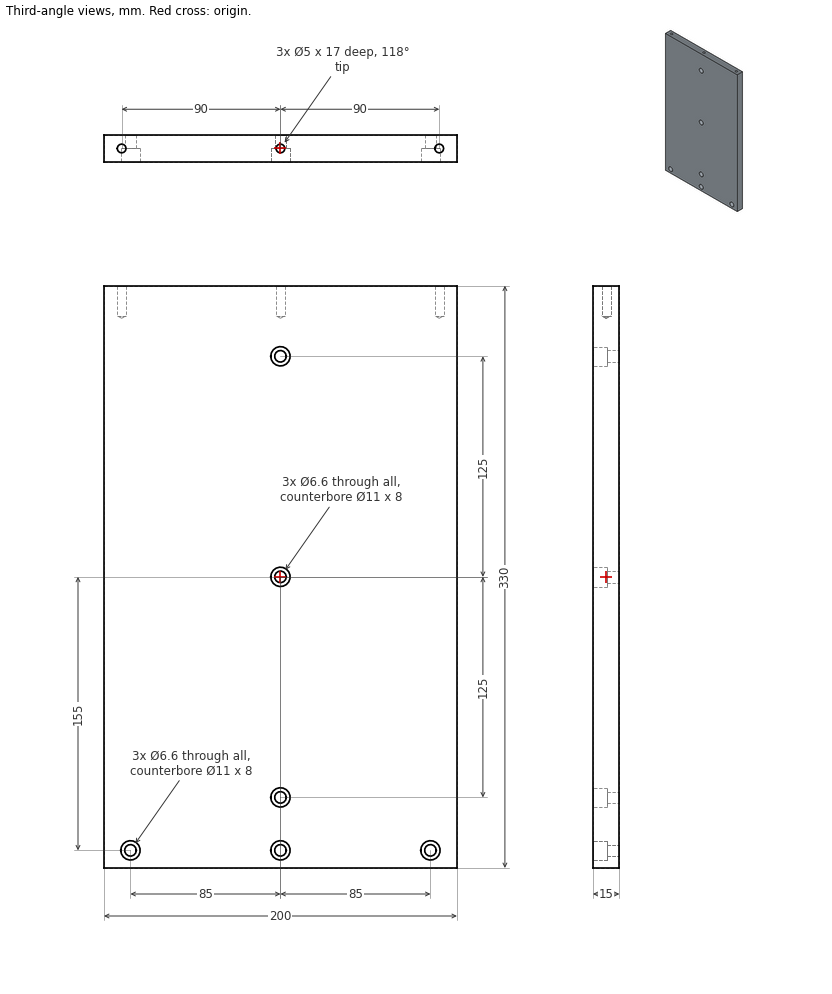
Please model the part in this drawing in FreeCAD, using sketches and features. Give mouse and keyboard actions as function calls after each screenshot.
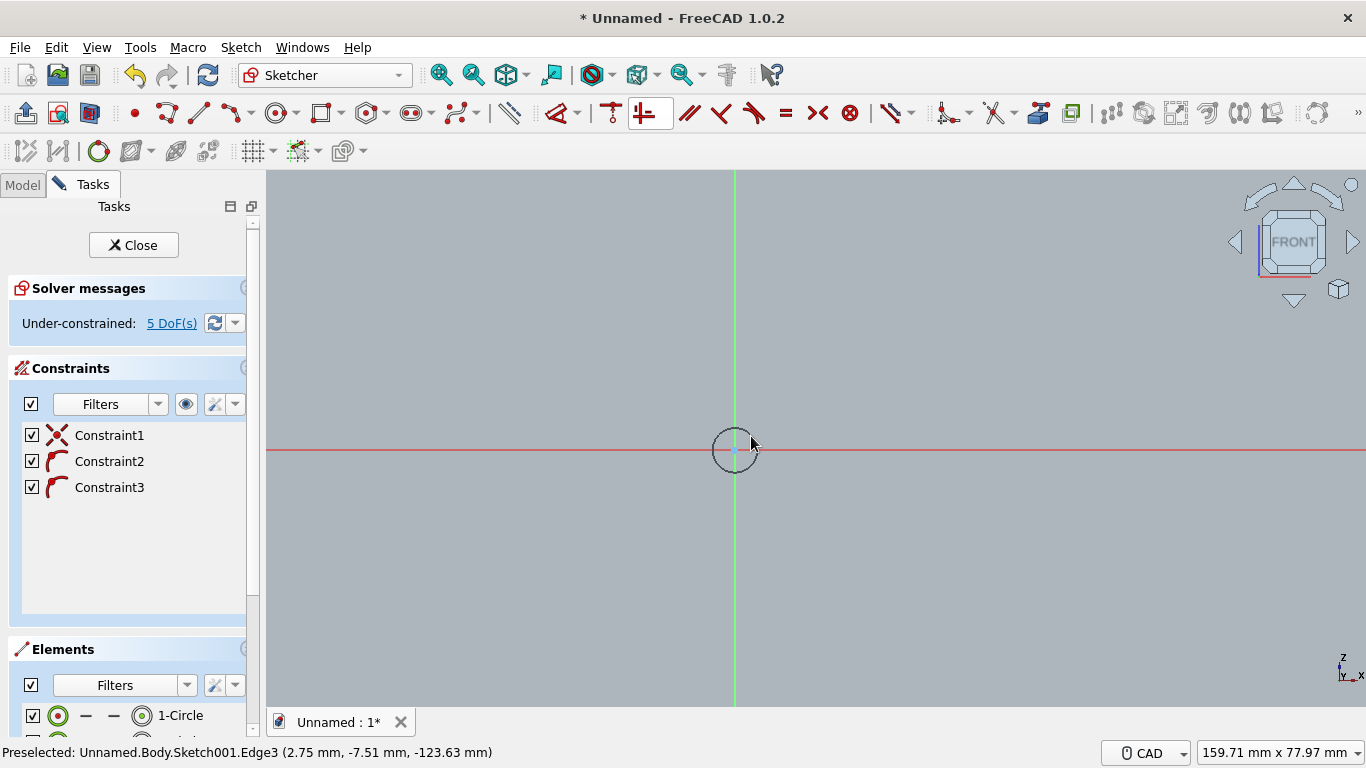
click(751, 435)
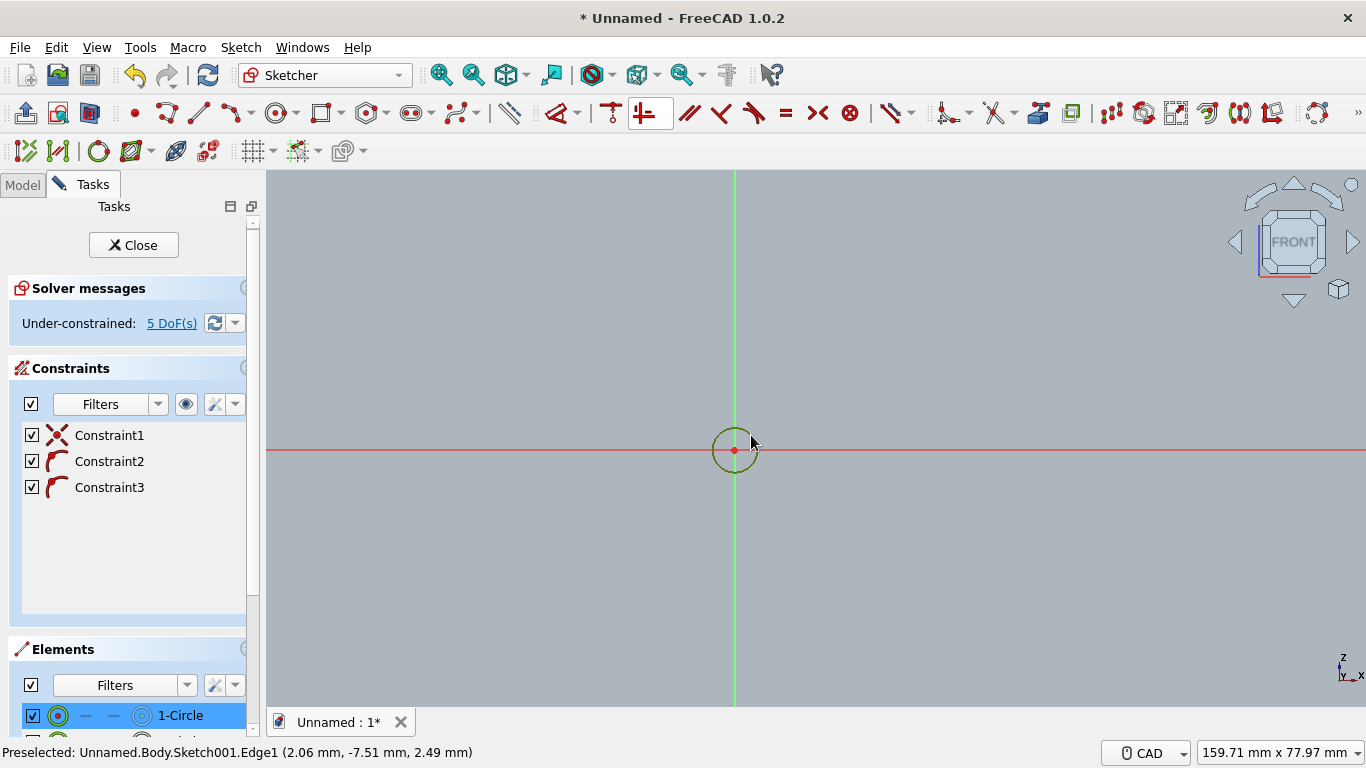
scroll(751, 435, down, 8)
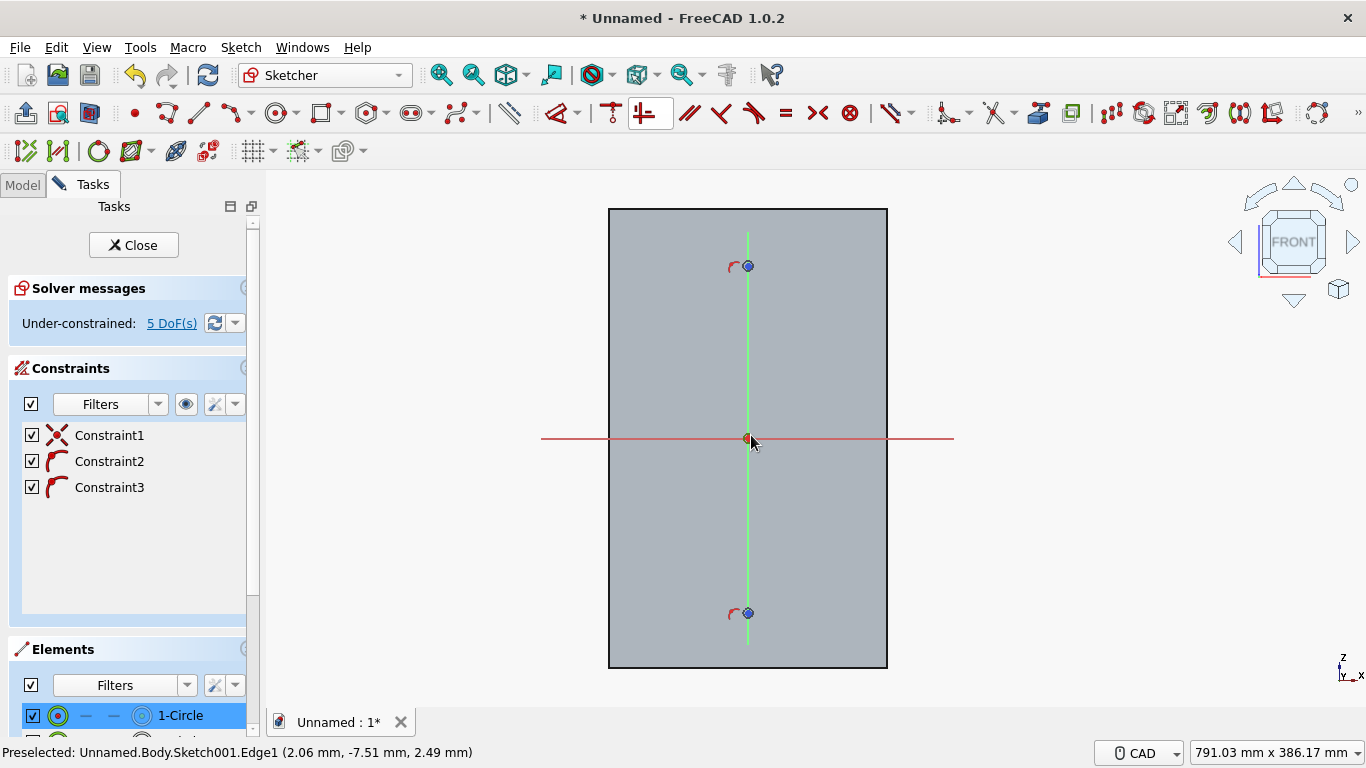
scroll(752, 262, up, 7)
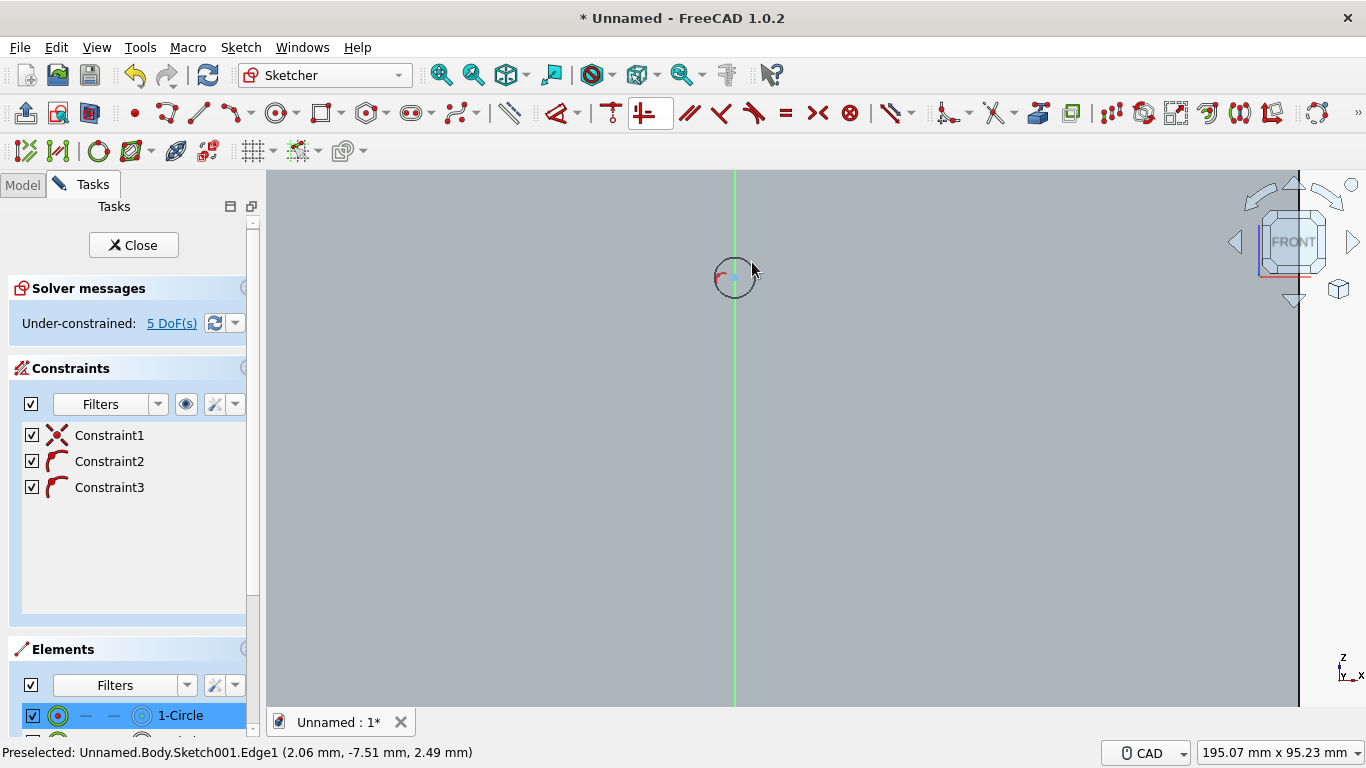
click(749, 263)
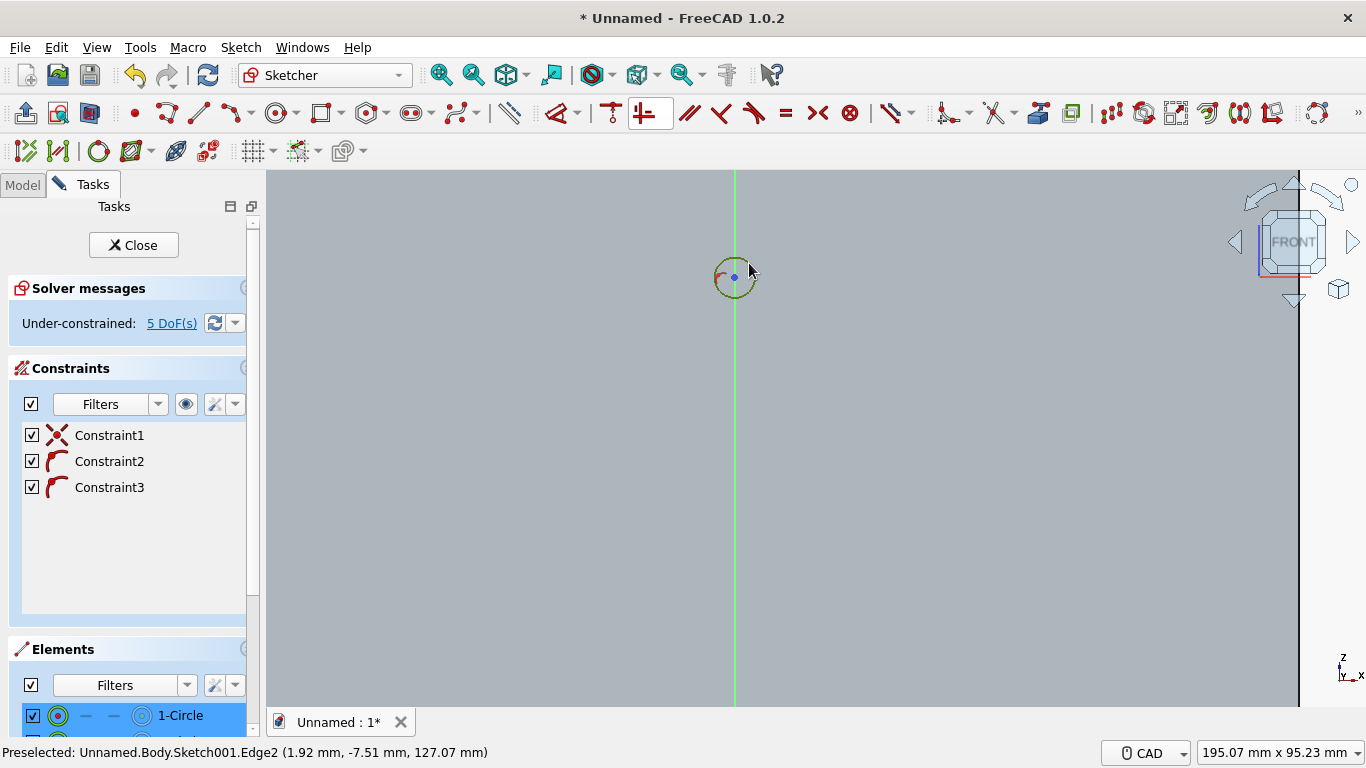
scroll(752, 262, down, 7)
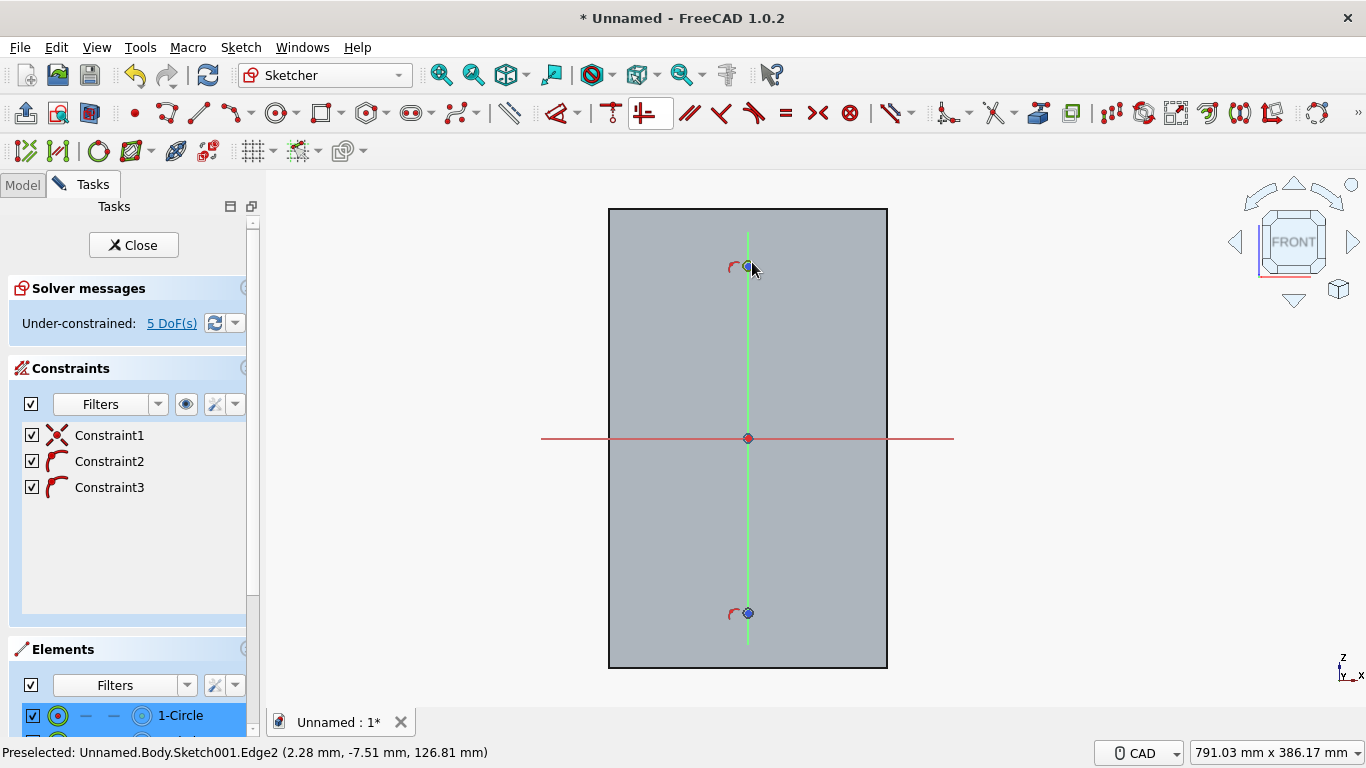
scroll(751, 610, up, 8)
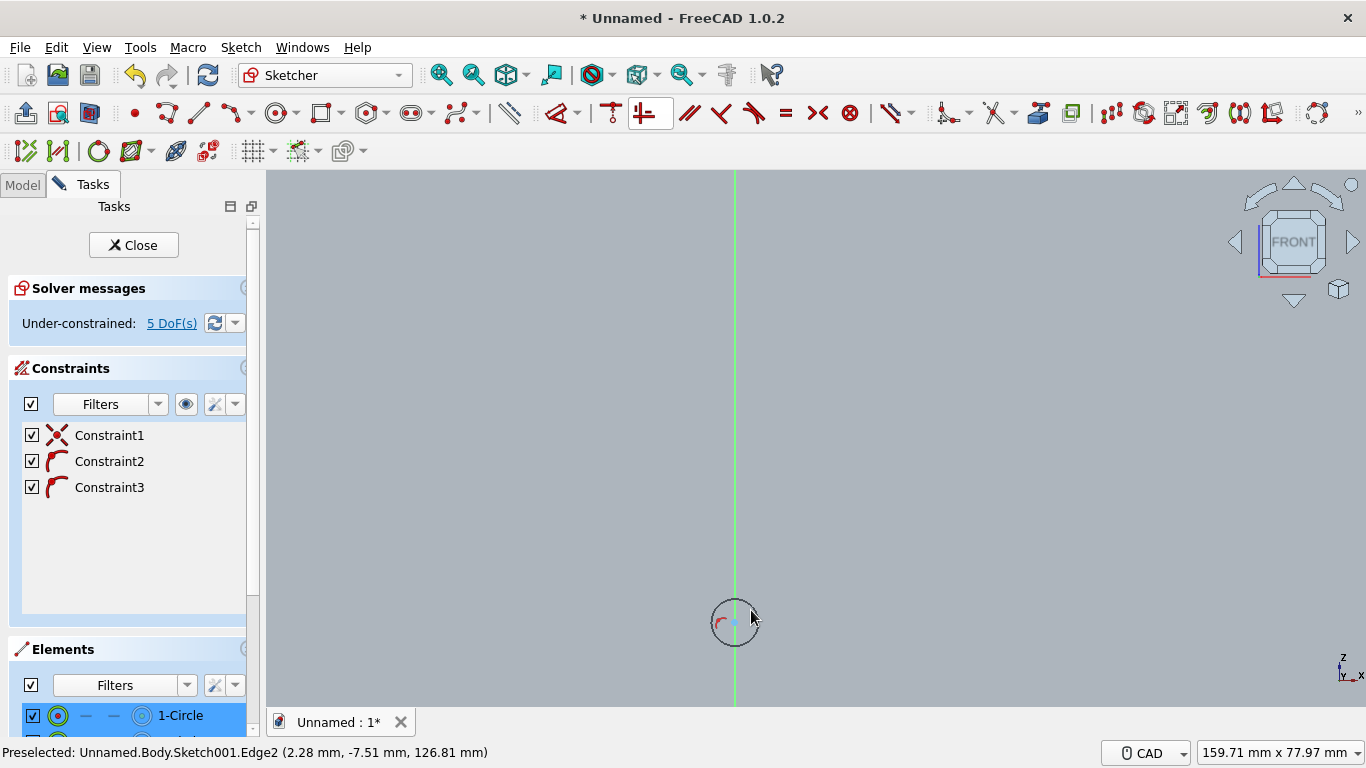
click(751, 606)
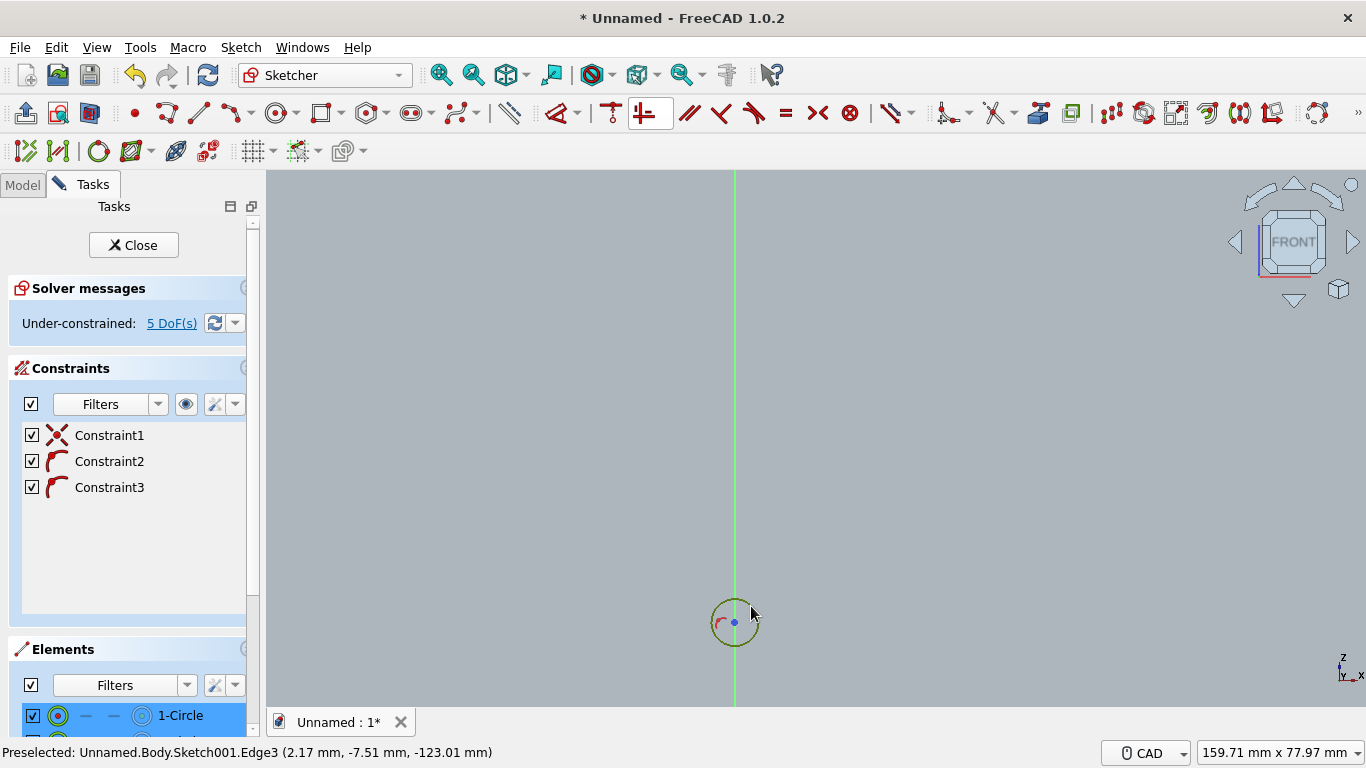
key(e)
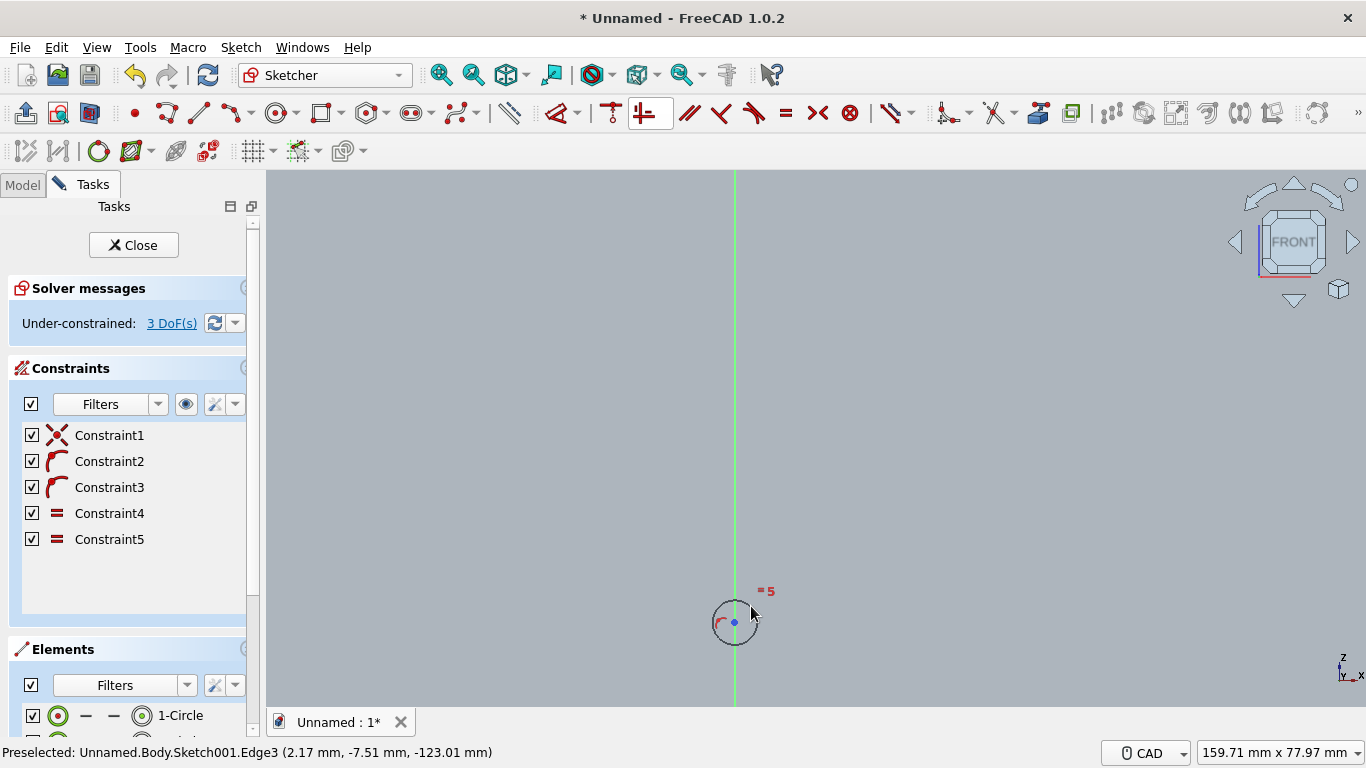
key(d)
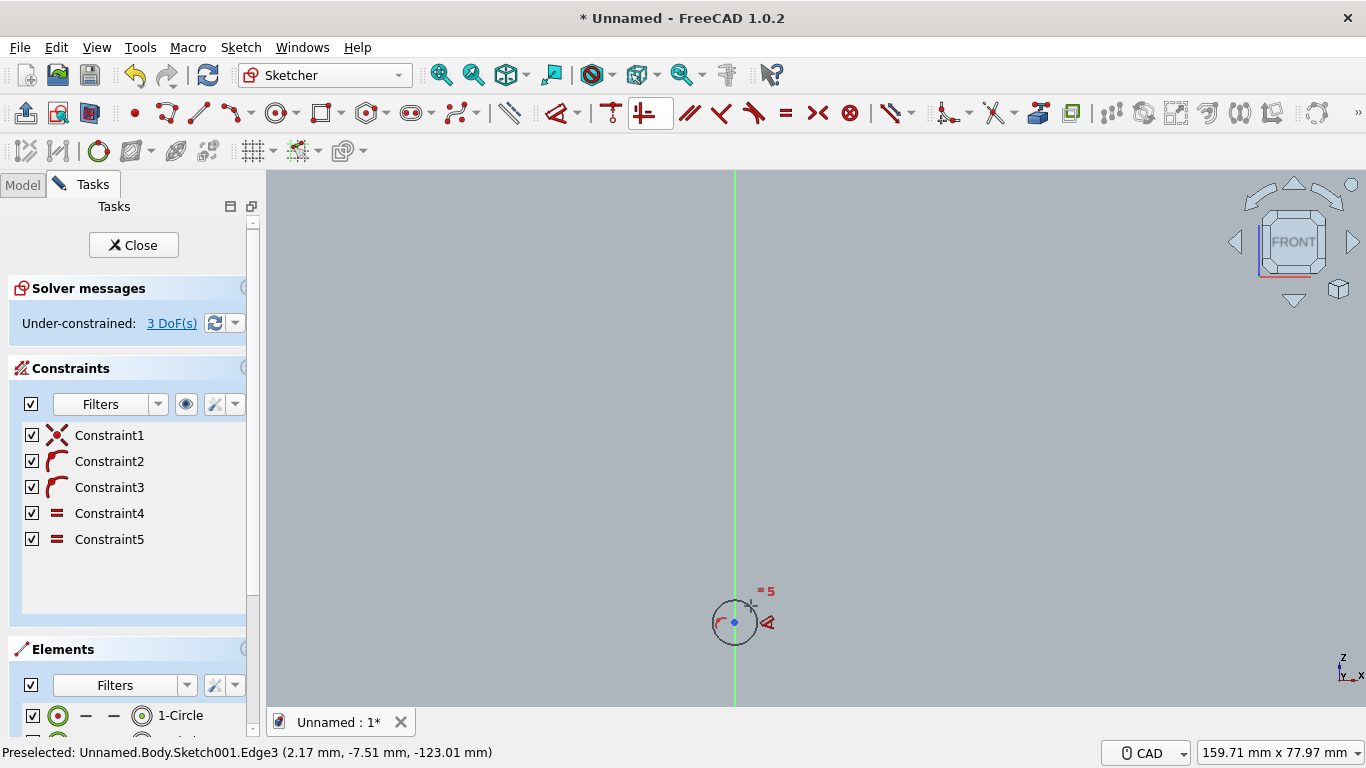
scroll(751, 611, down, 8)